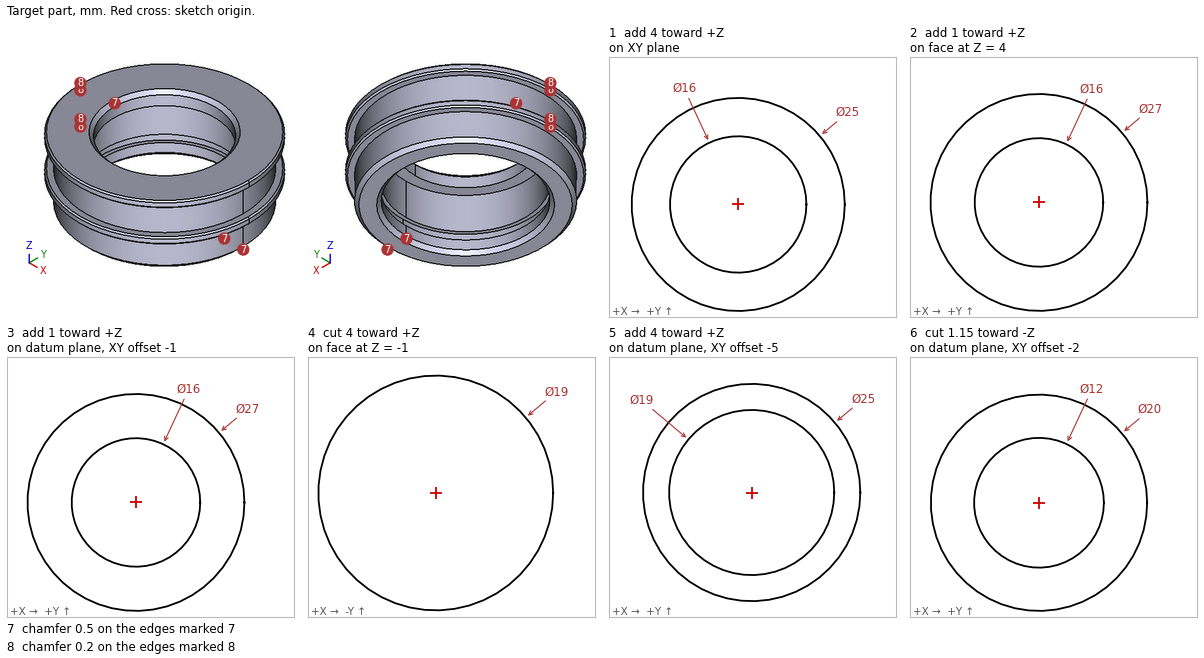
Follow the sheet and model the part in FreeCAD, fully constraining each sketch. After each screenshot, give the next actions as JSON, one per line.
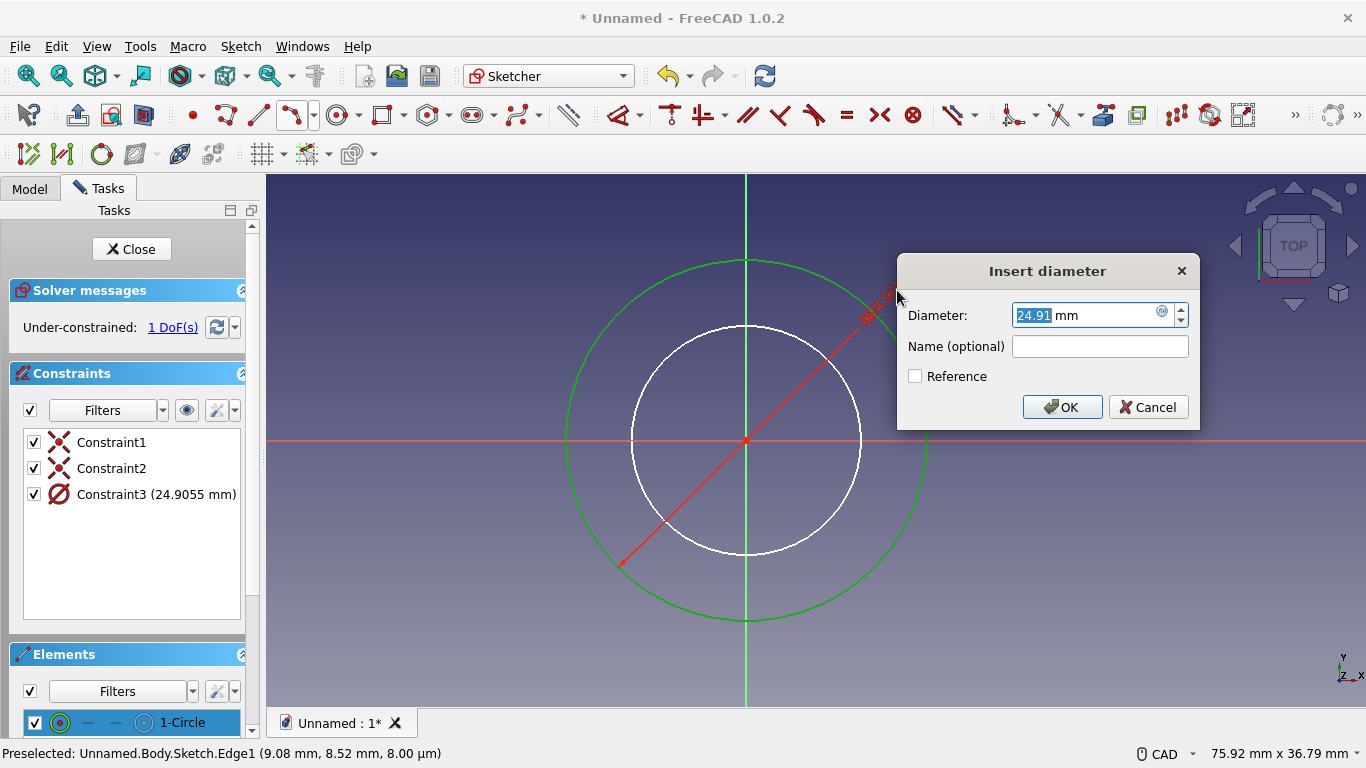
{"action": "type", "text": "25"}
{"action": "key", "text": "Return"}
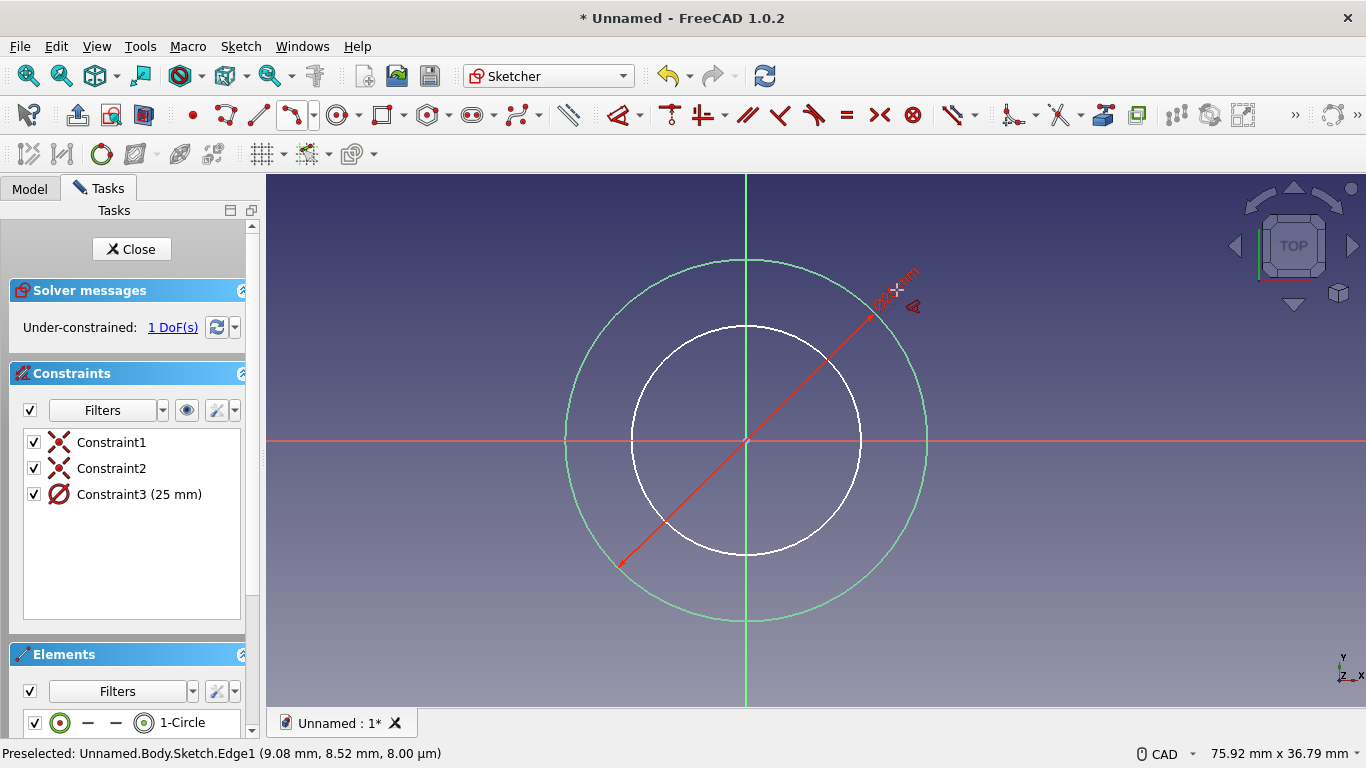
{"action": "left_click", "coordinate": [827, 359]}
{"action": "left_click", "coordinate": [850, 336]}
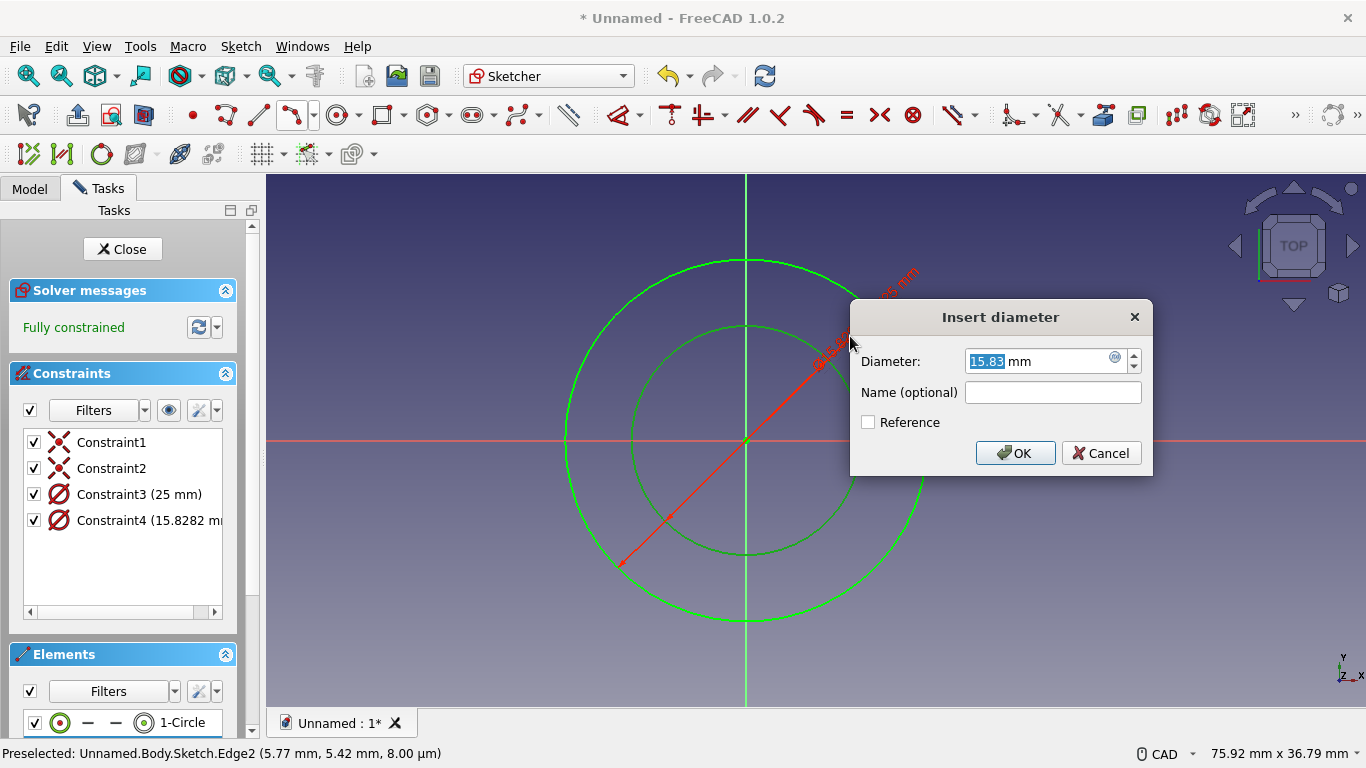
{"action": "type", "text": "16"}
{"action": "key", "text": "Return"}
{"action": "key", "text": "Escape"}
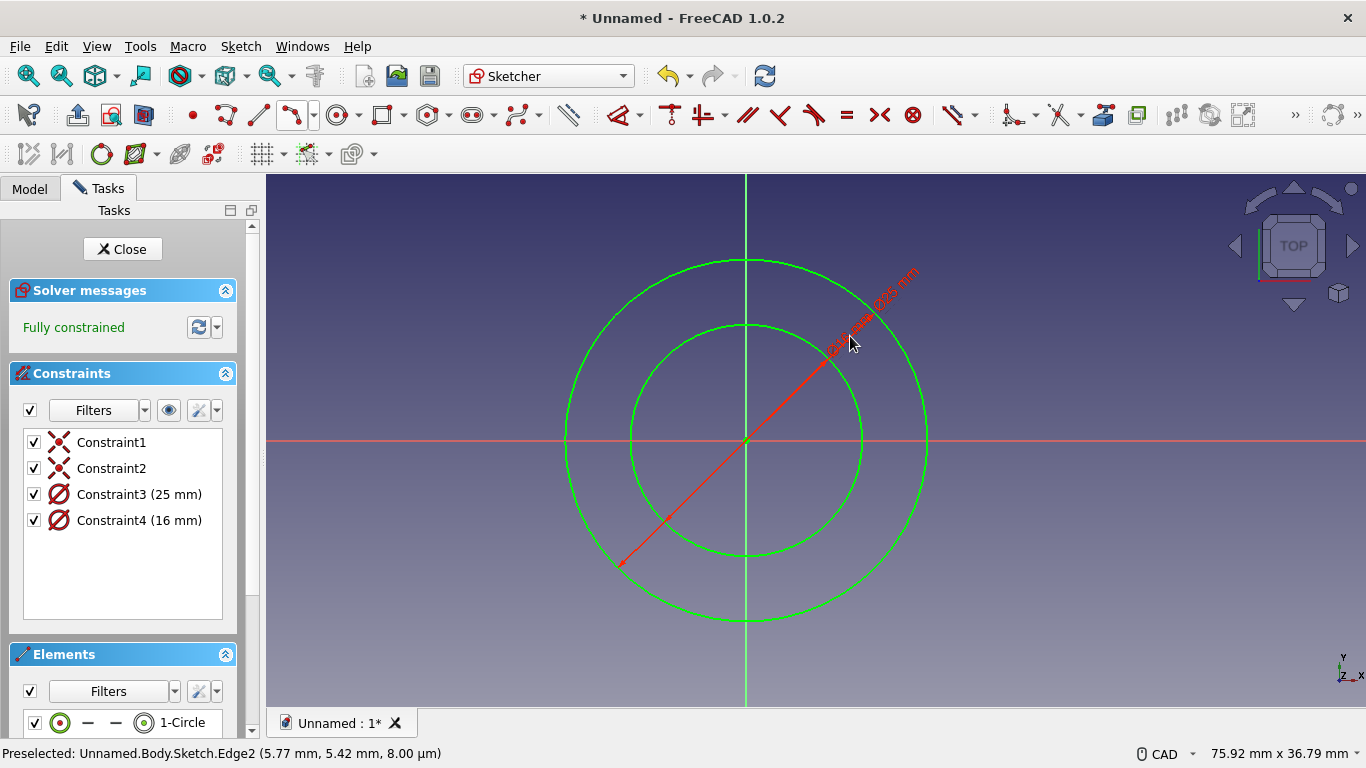
{"action": "left_click", "coordinate": [123, 249]}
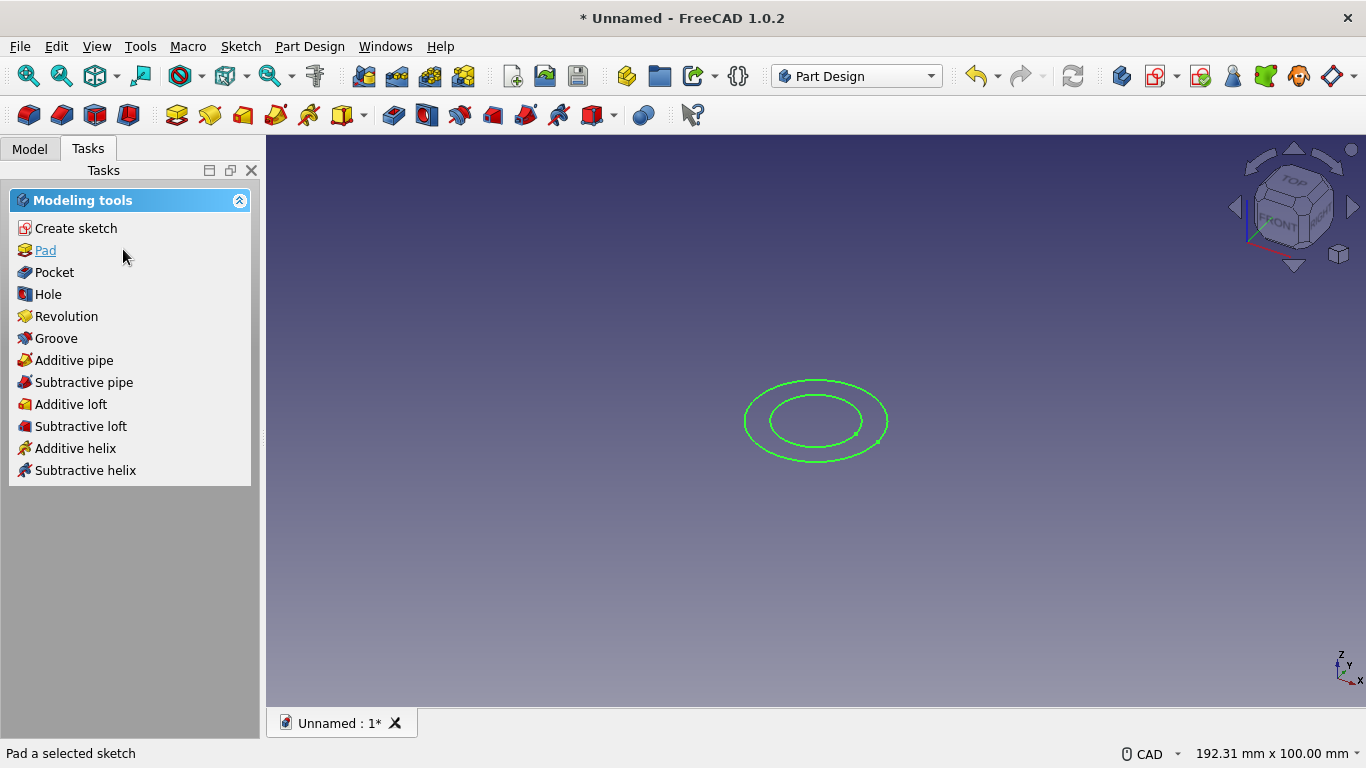
{"action": "left_click", "coordinate": [177, 116]}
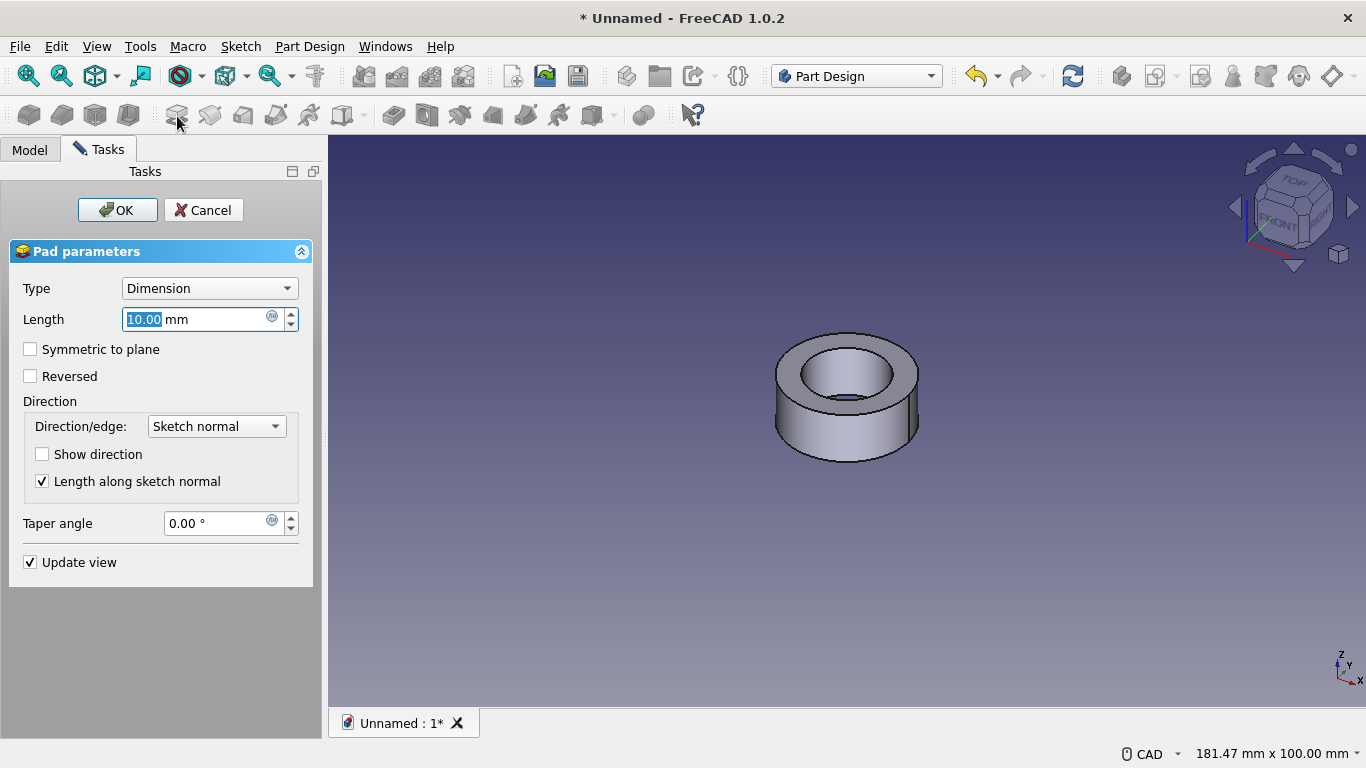
{"action": "type", "text": "4"}
{"action": "key", "text": "Tab"}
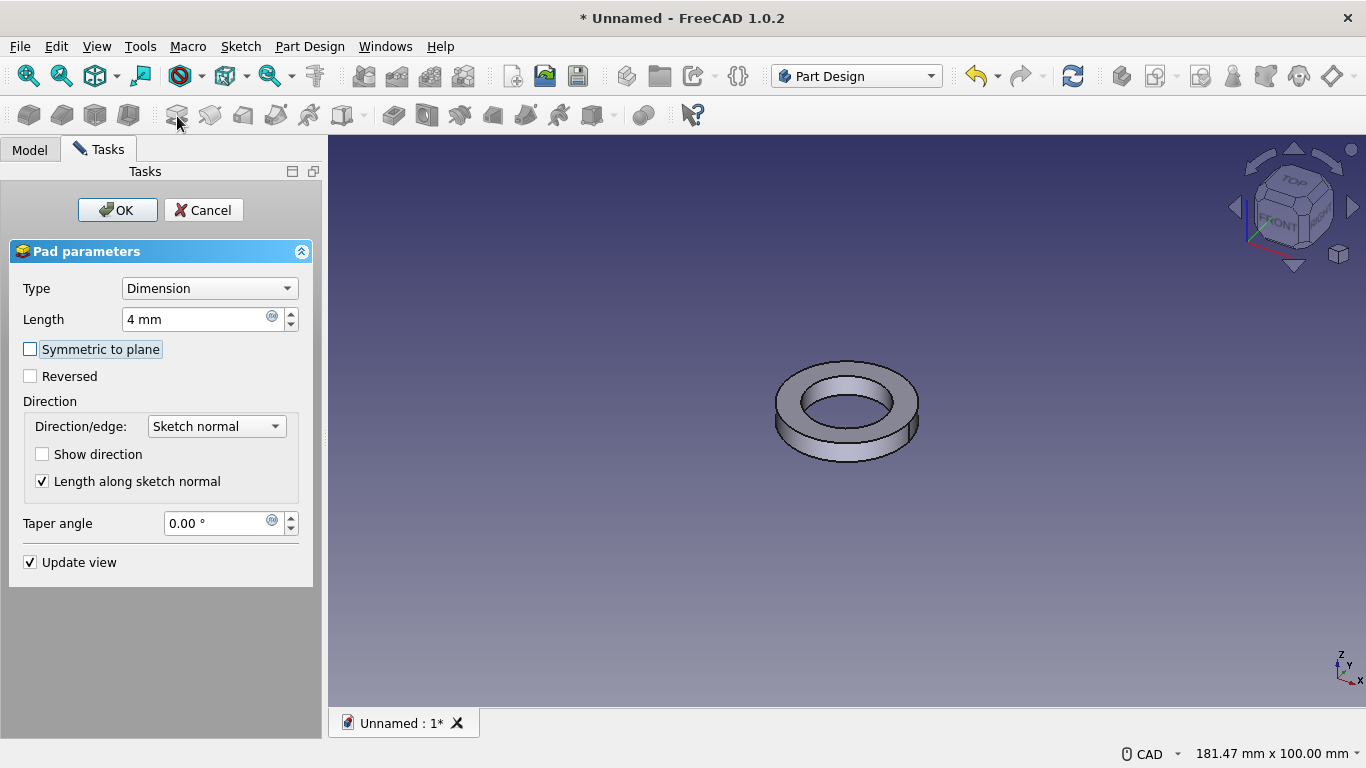
{"action": "left_click", "coordinate": [118, 210]}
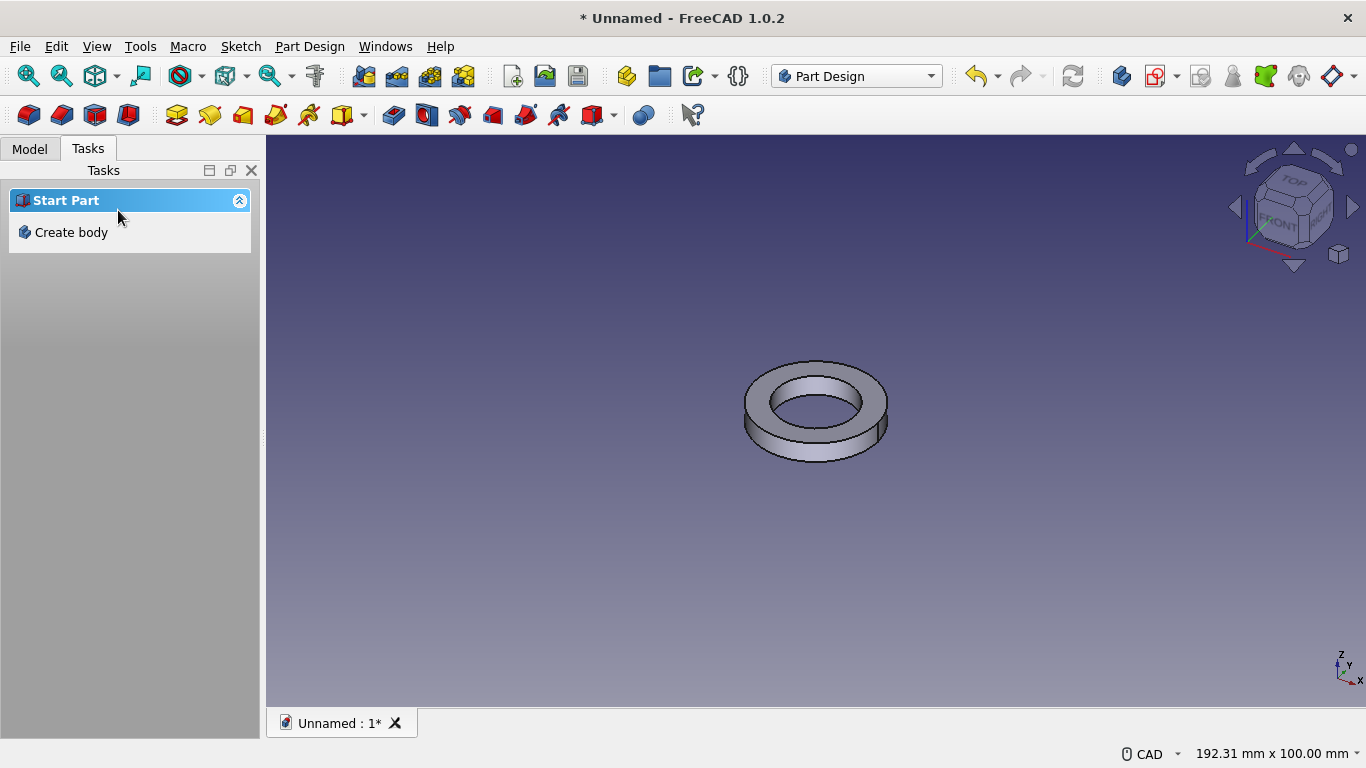
{"action": "left_click", "coordinate": [29, 76]}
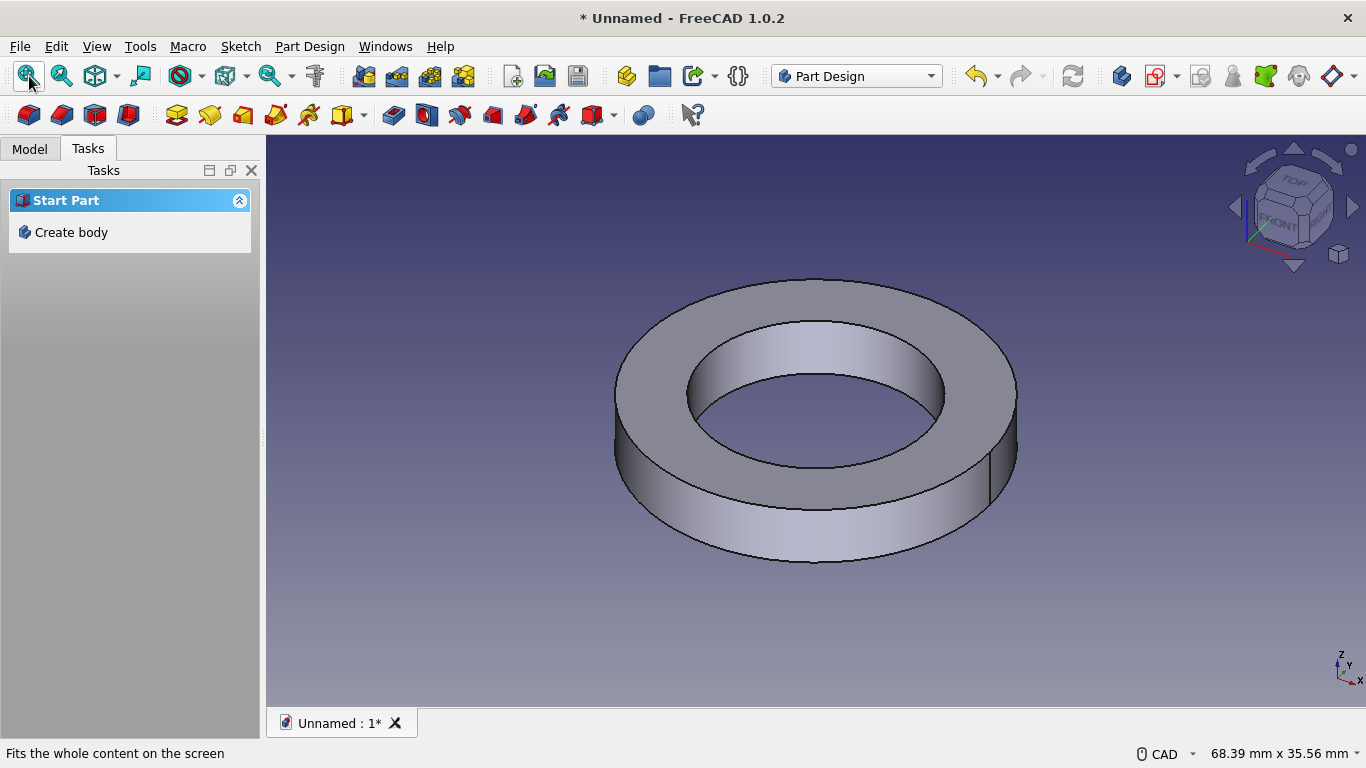
{"action": "left_click", "coordinate": [774, 304]}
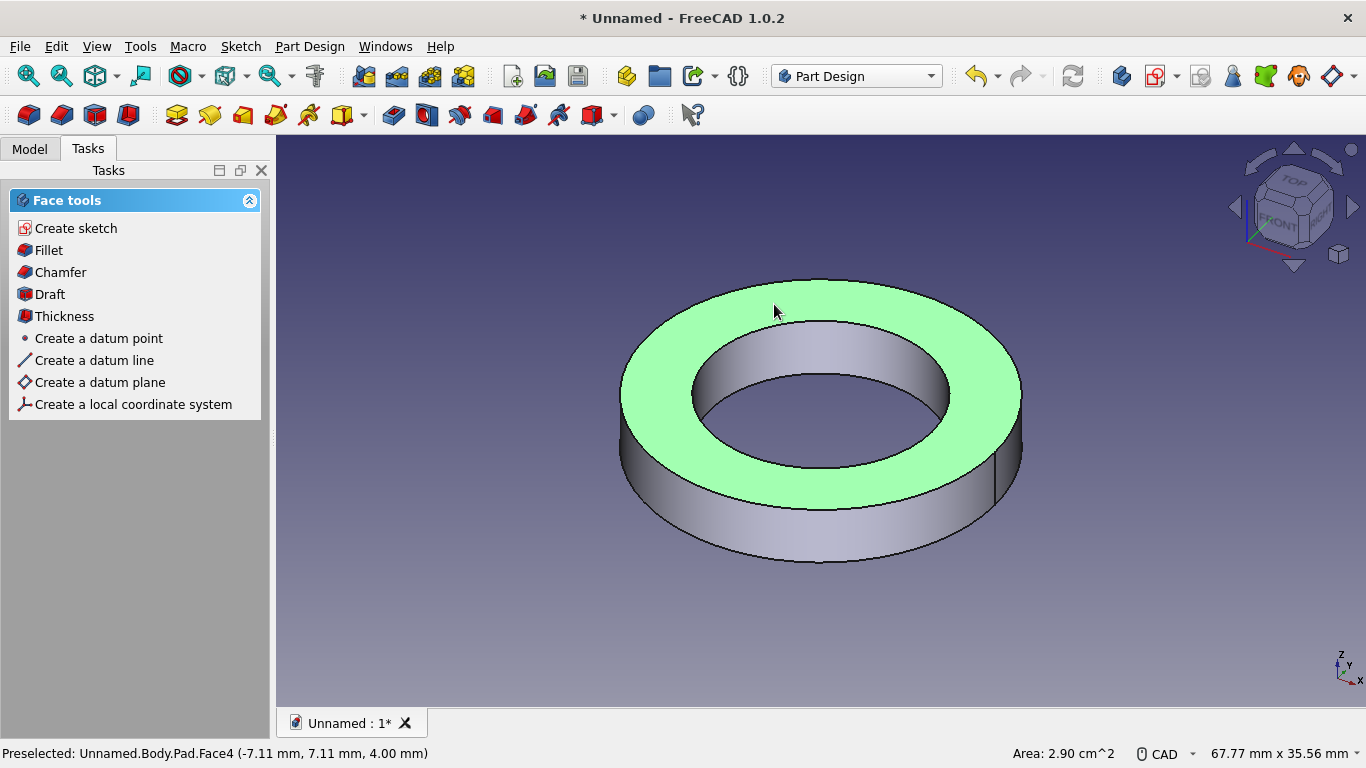
{"action": "left_click", "coordinate": [1154, 76]}